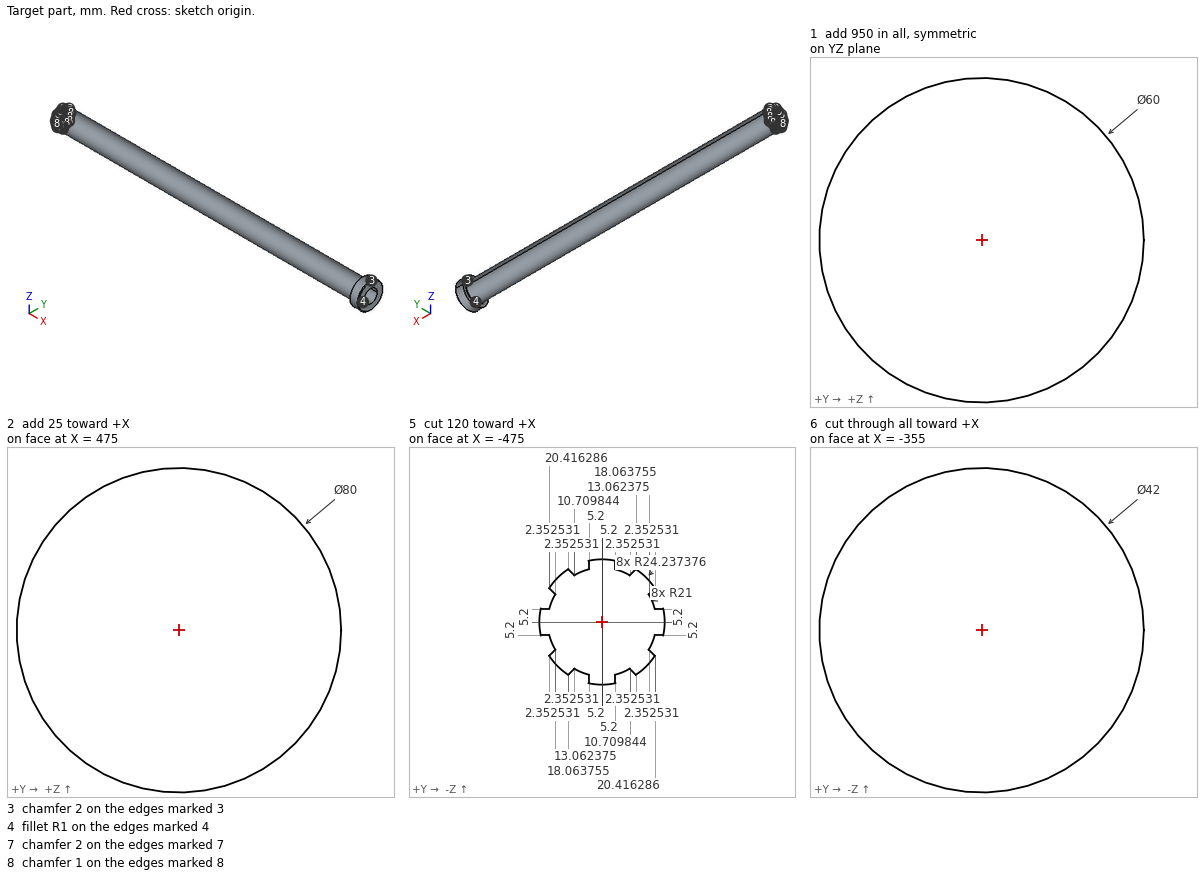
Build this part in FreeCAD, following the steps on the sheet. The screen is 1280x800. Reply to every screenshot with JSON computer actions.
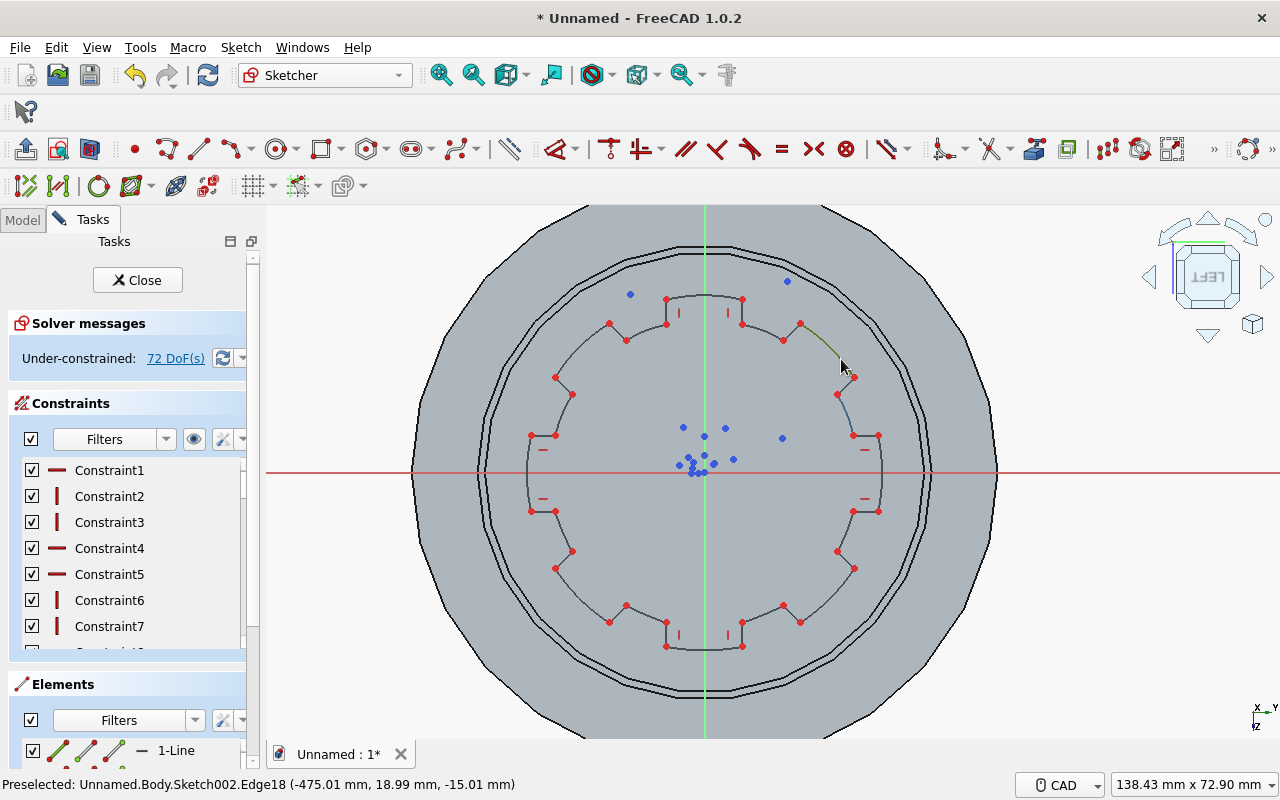
{"action": "key", "text": "c"}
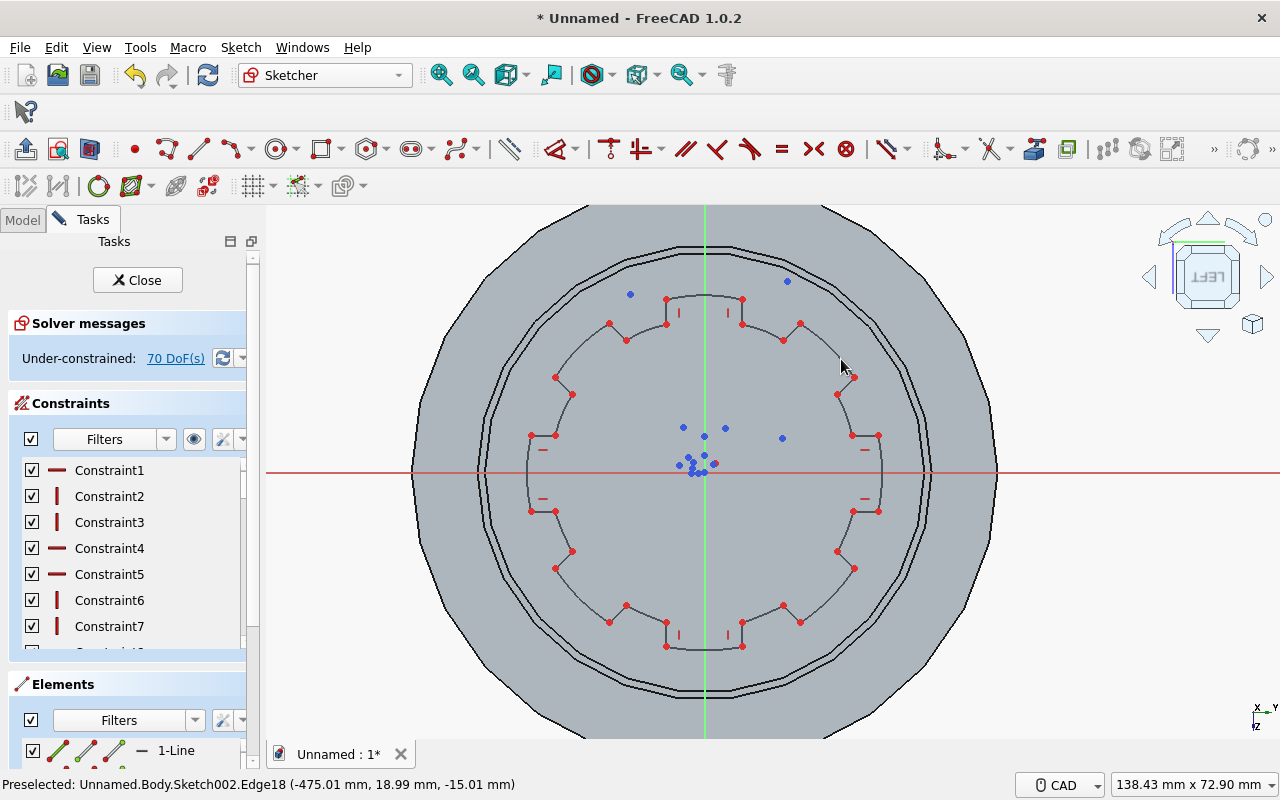
{"action": "left_click", "coordinate": [849, 423]}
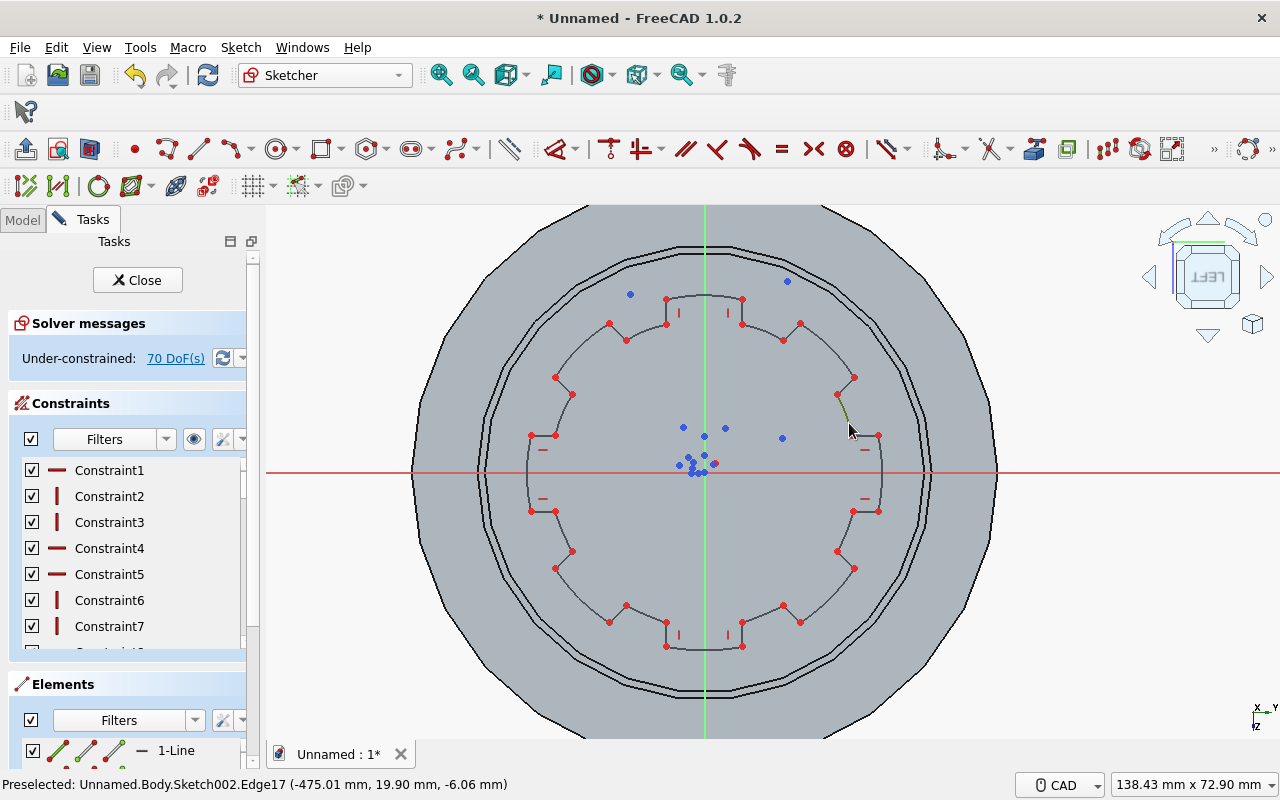
{"action": "left_click", "coordinate": [772, 334]}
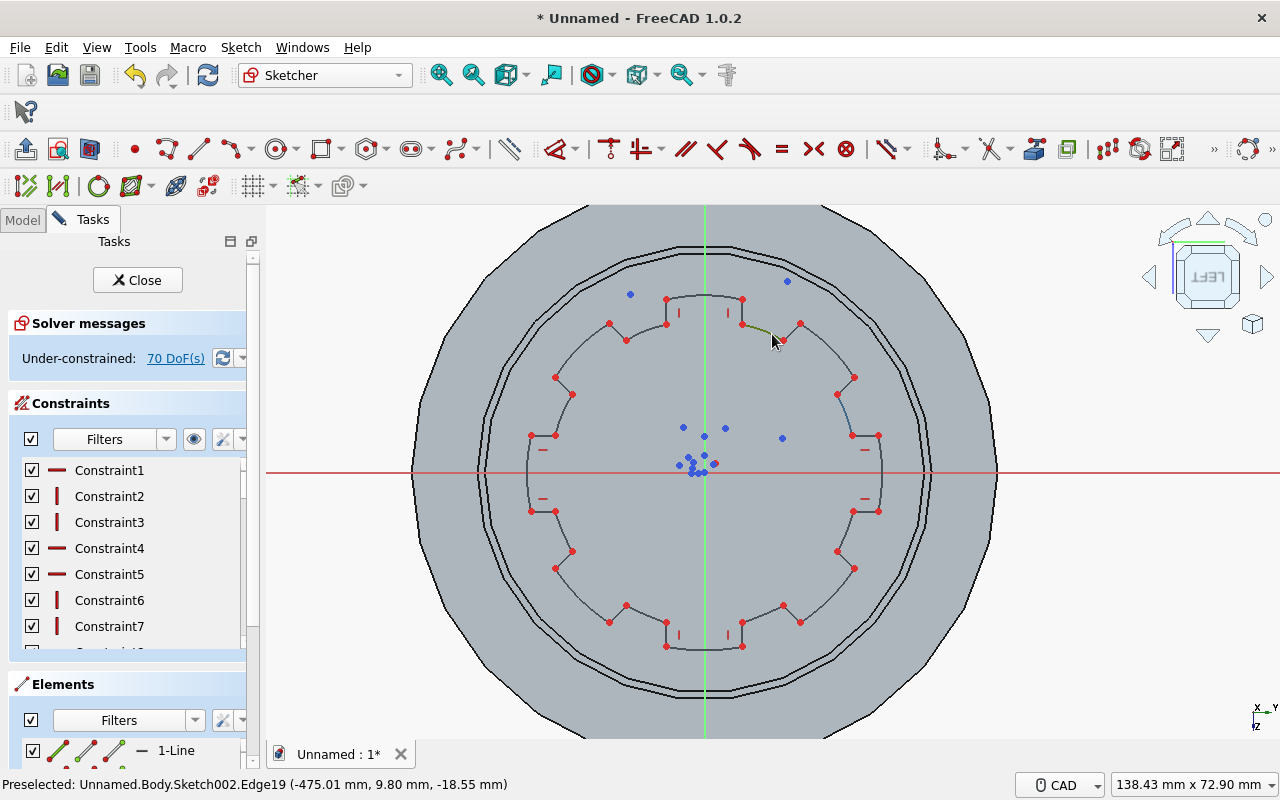
{"action": "key", "text": "c"}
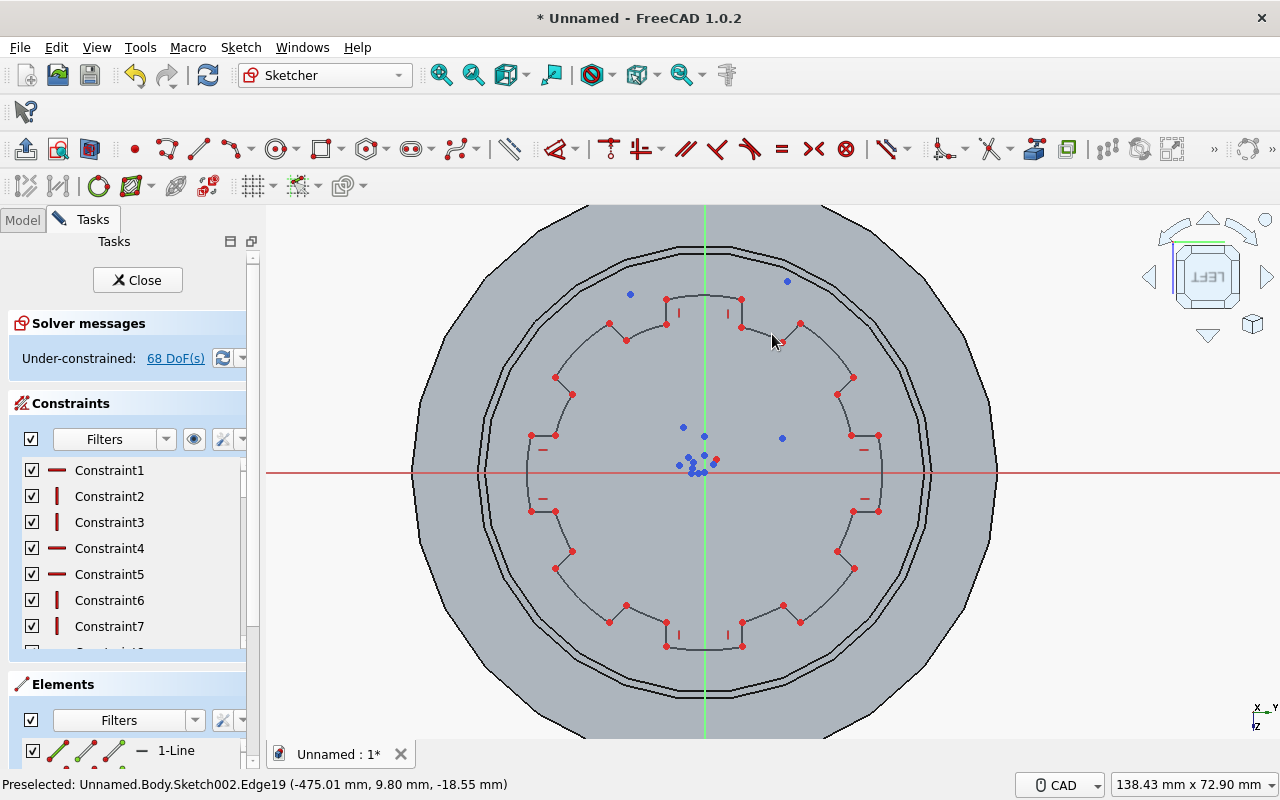
{"action": "left_click", "coordinate": [848, 423]}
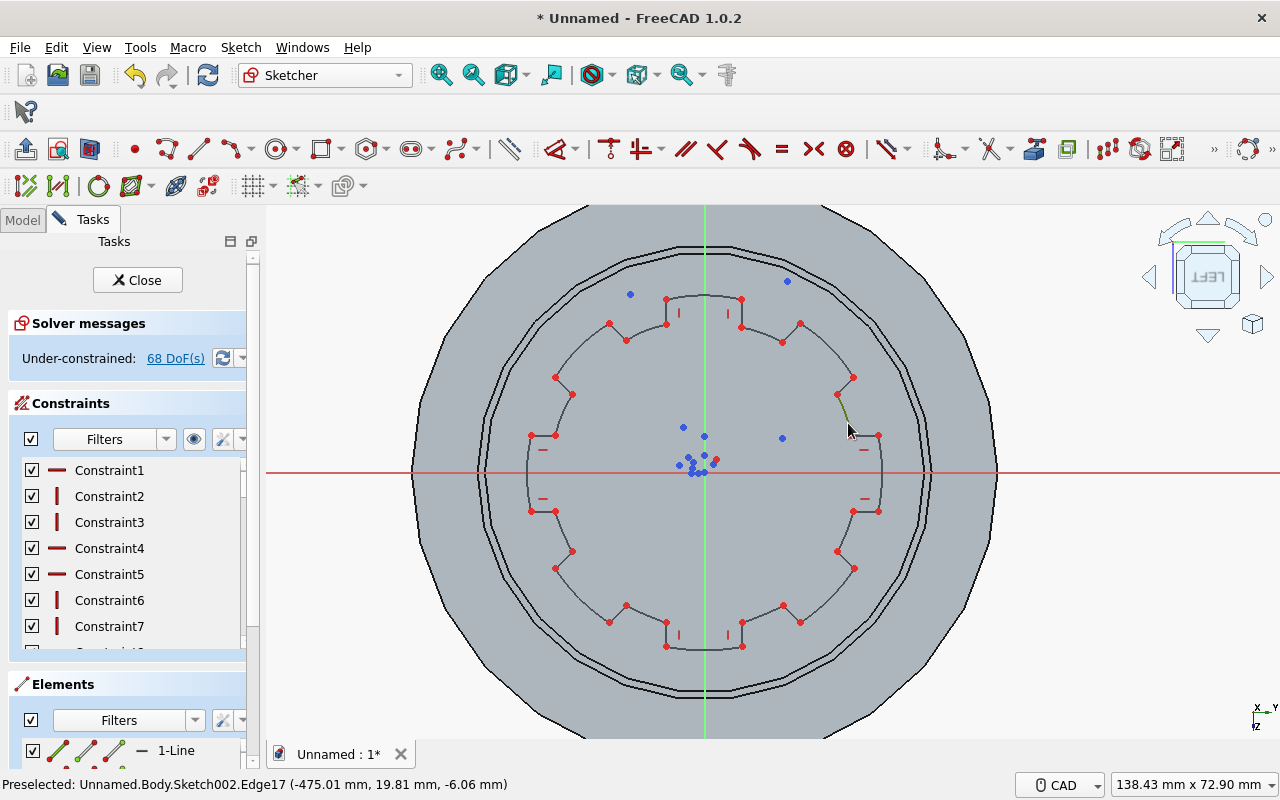
{"action": "left_click", "coordinate": [719, 296]}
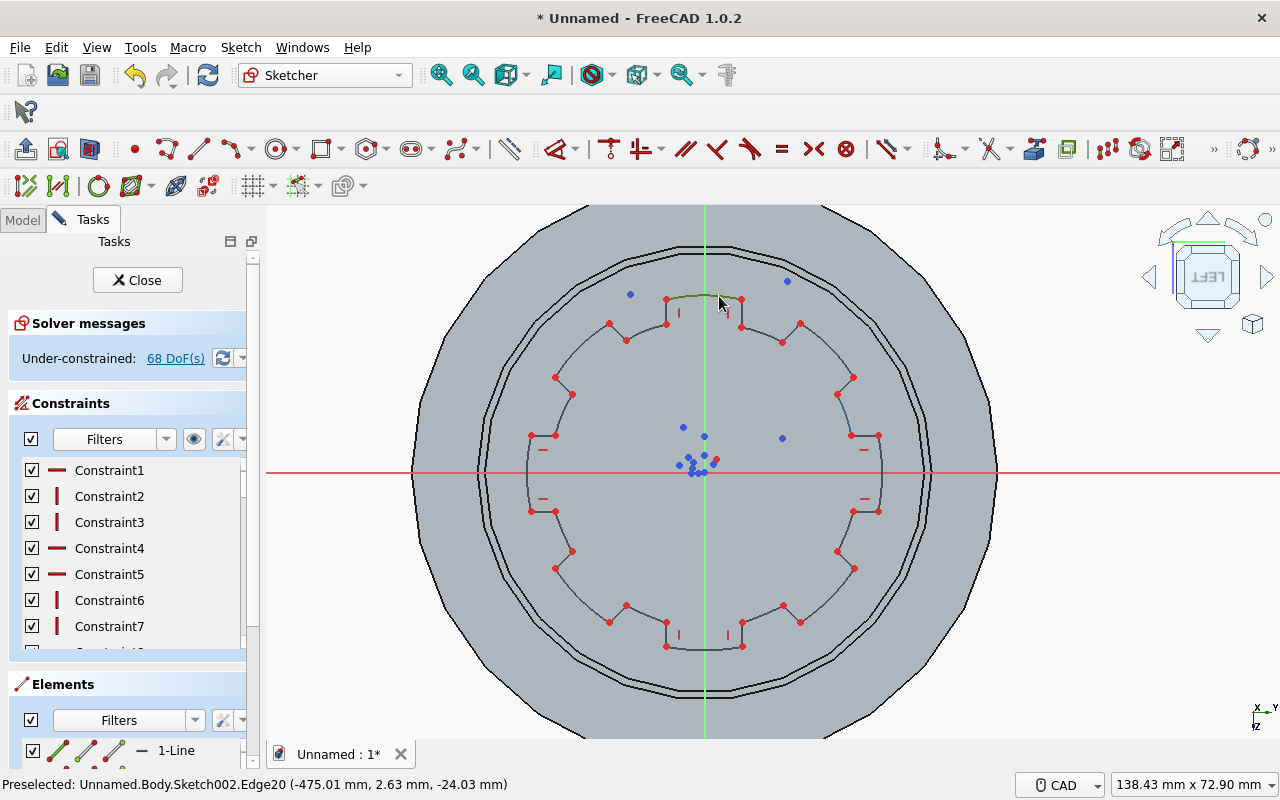
{"action": "key", "text": "c"}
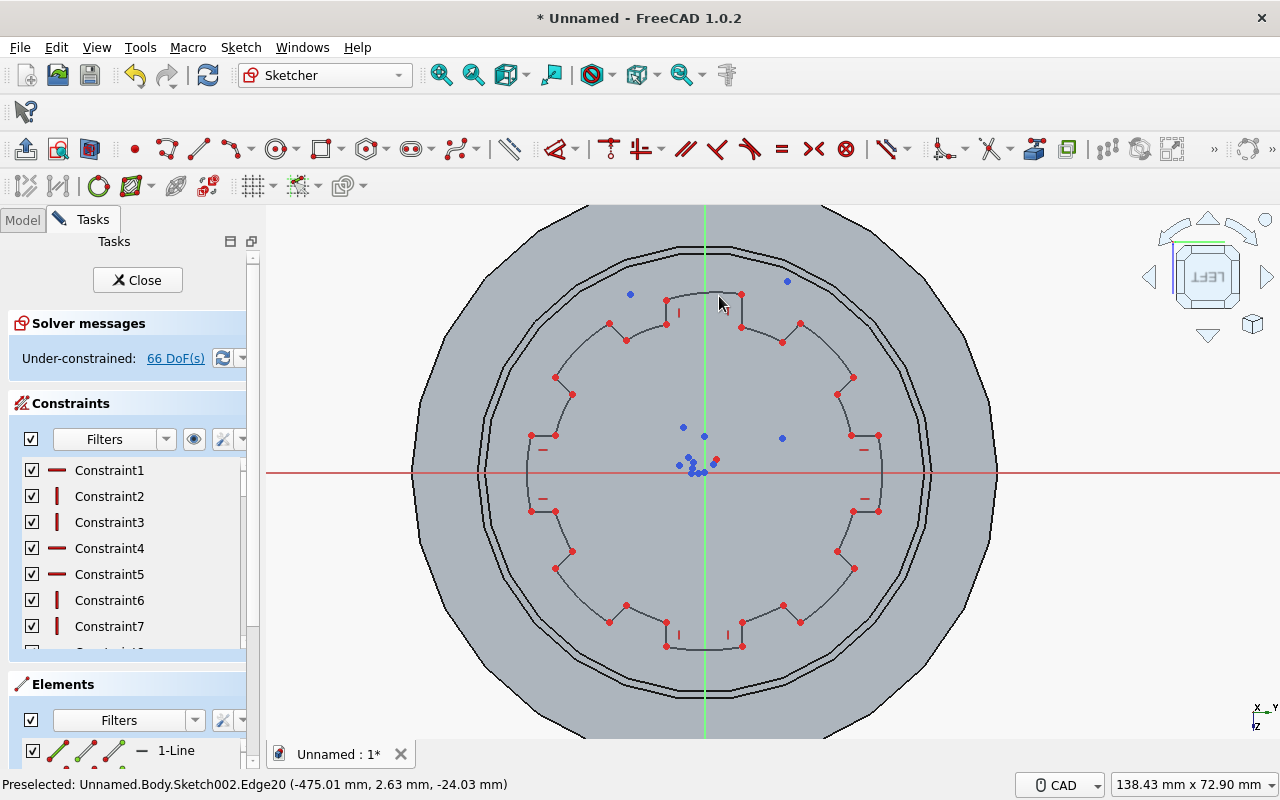
{"action": "left_click", "coordinate": [848, 423]}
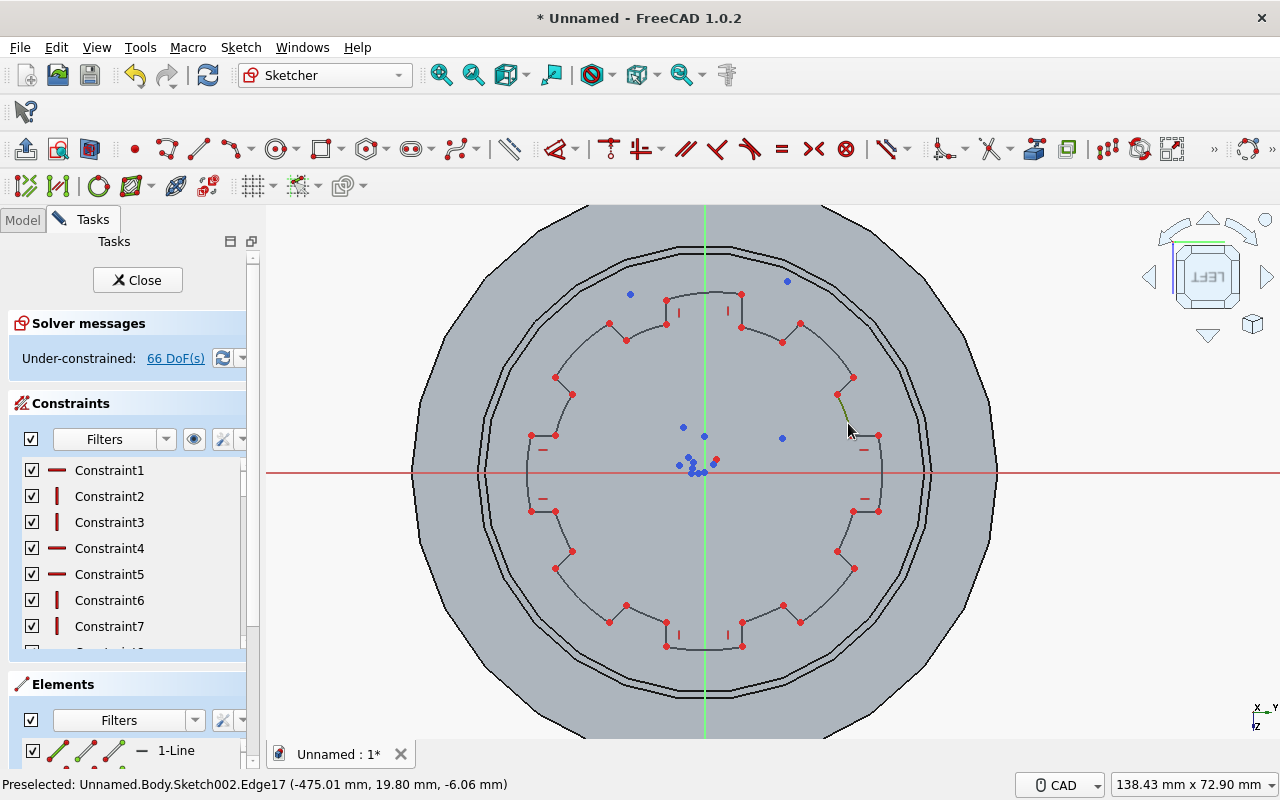
{"action": "left_click", "coordinate": [654, 328]}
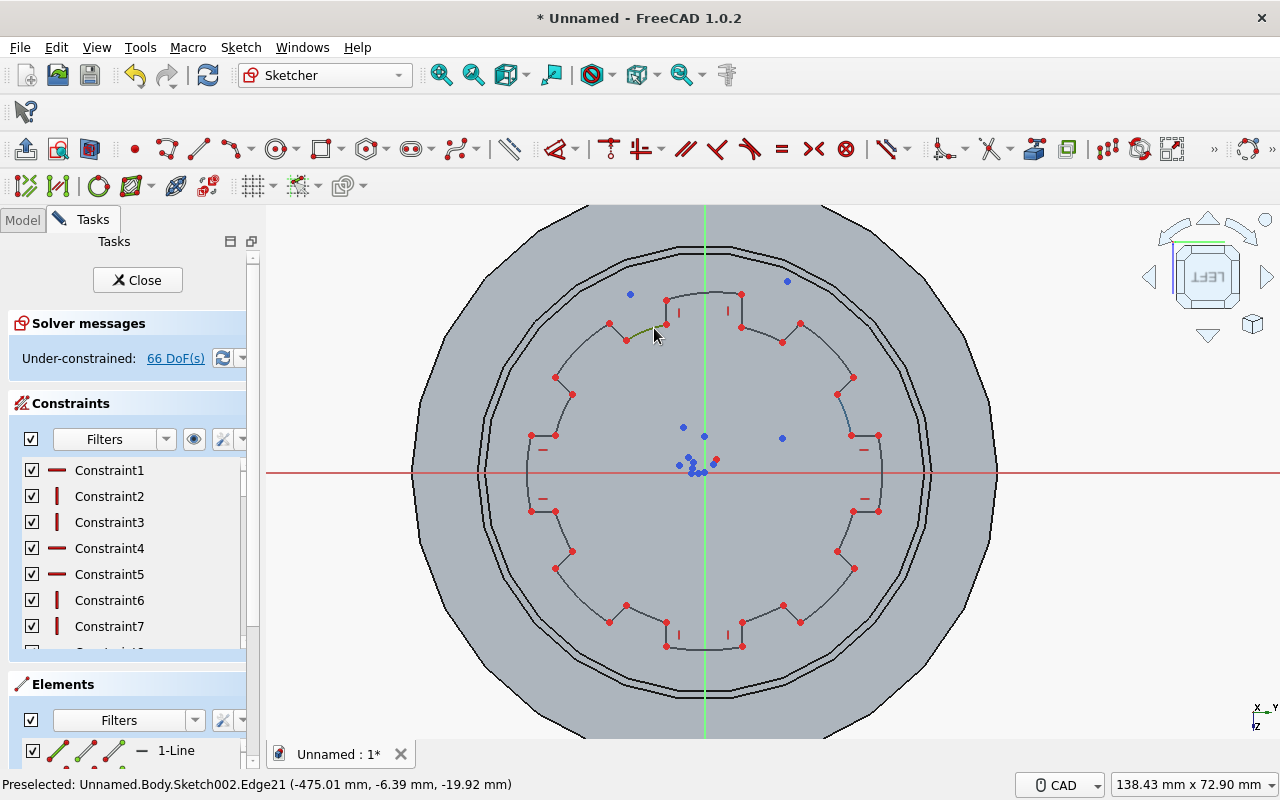
{"action": "left_click", "coordinate": [610, 150]}